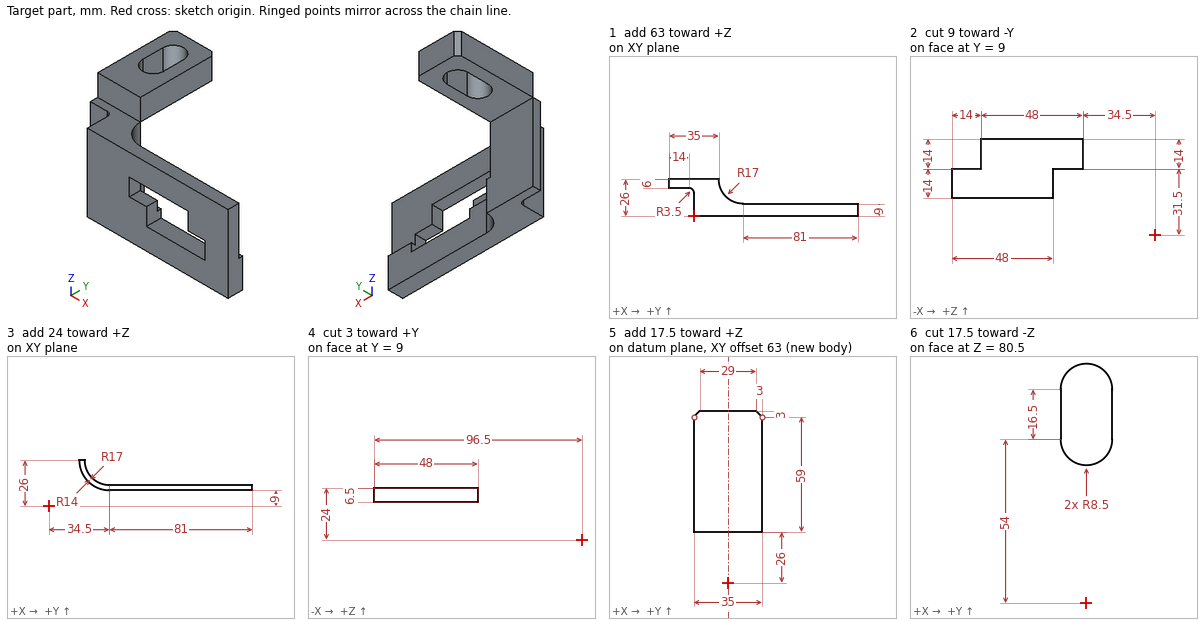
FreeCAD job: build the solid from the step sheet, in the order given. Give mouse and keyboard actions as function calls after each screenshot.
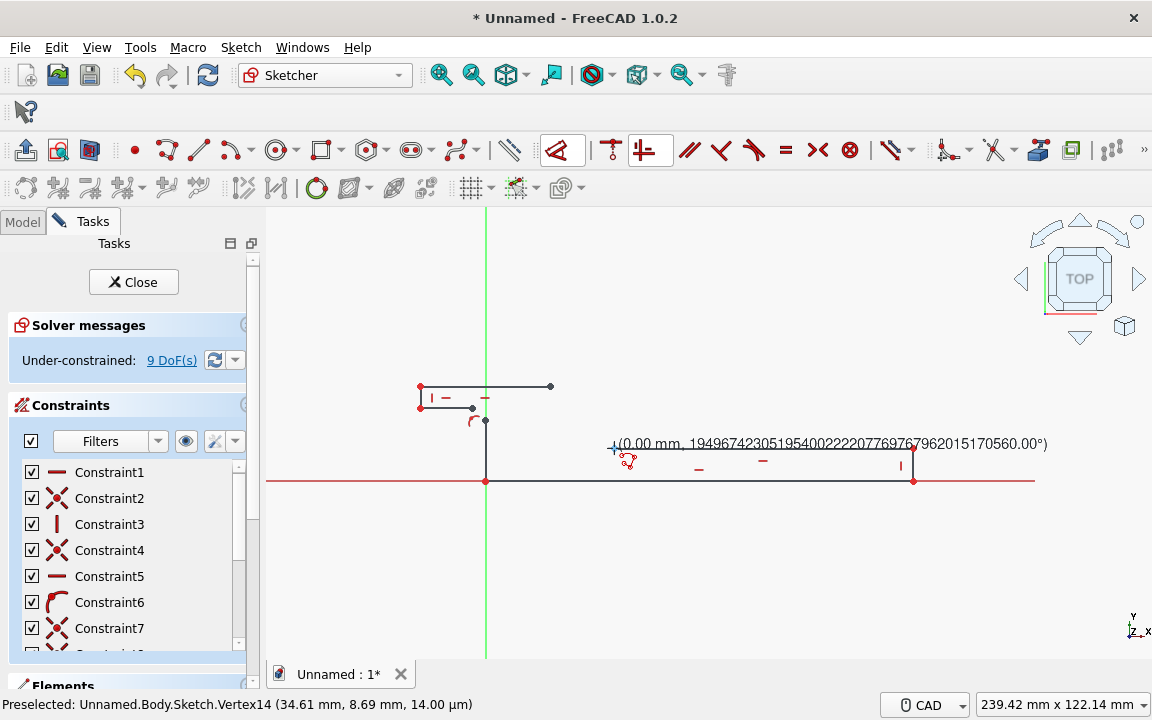
key(g)
key(3)
key(a)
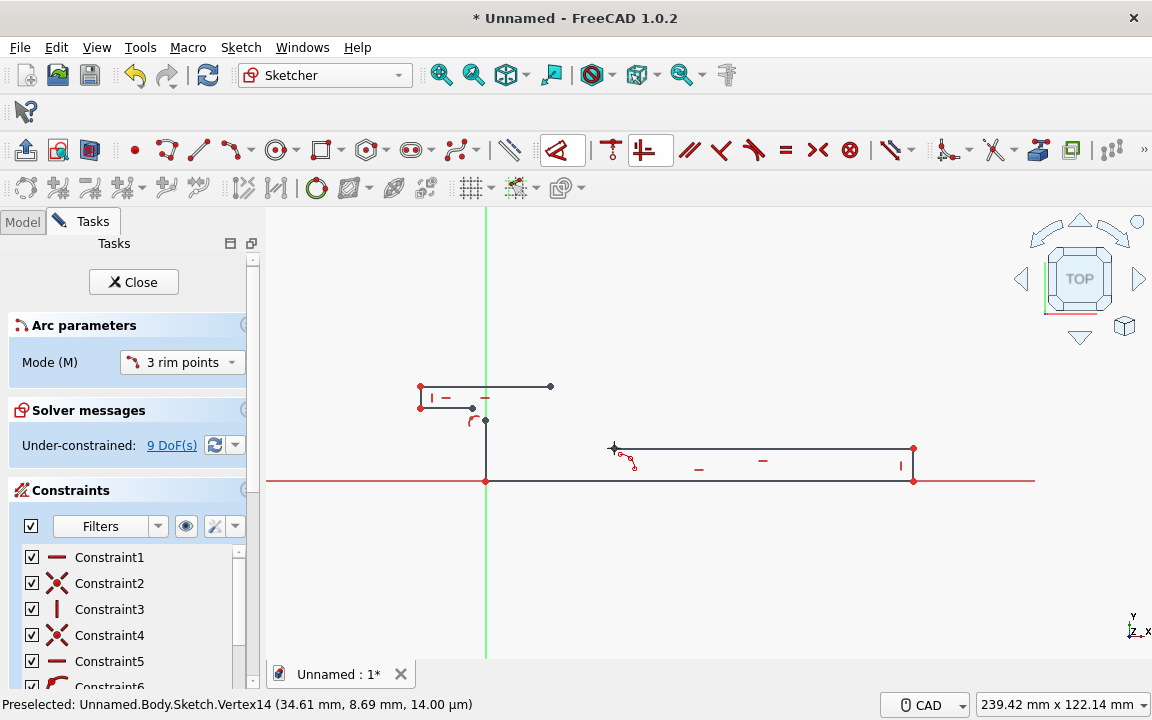
scroll(473, 407, up, 2)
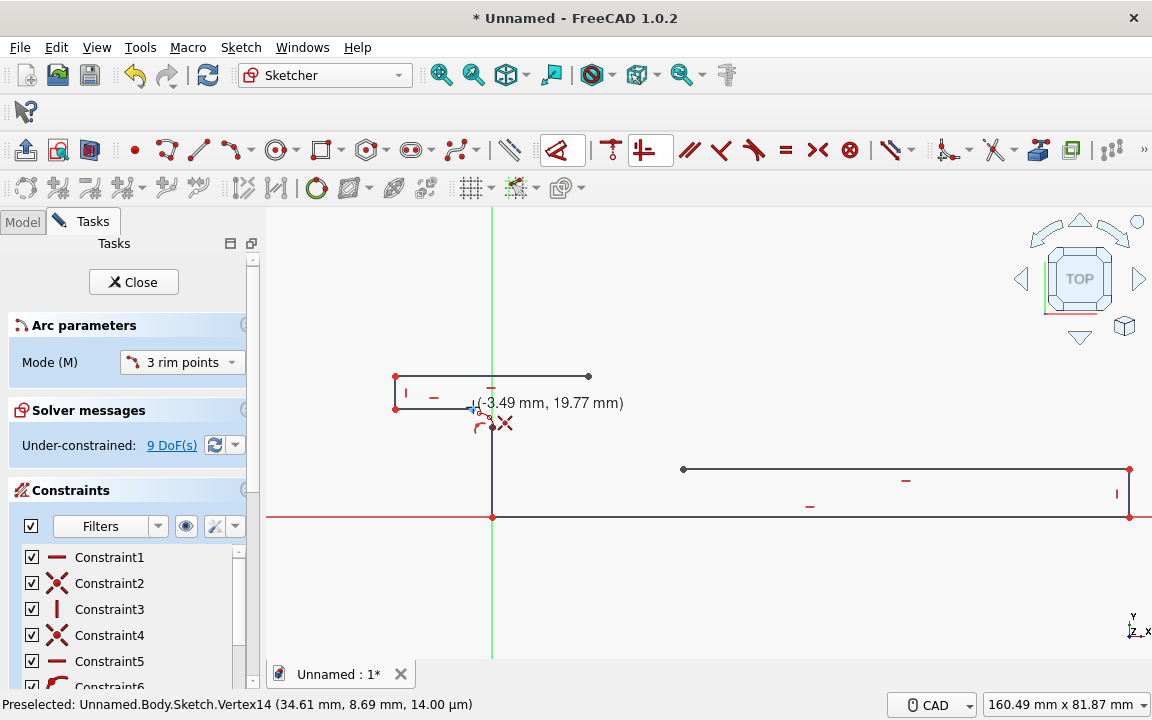
click(473, 409)
click(492, 428)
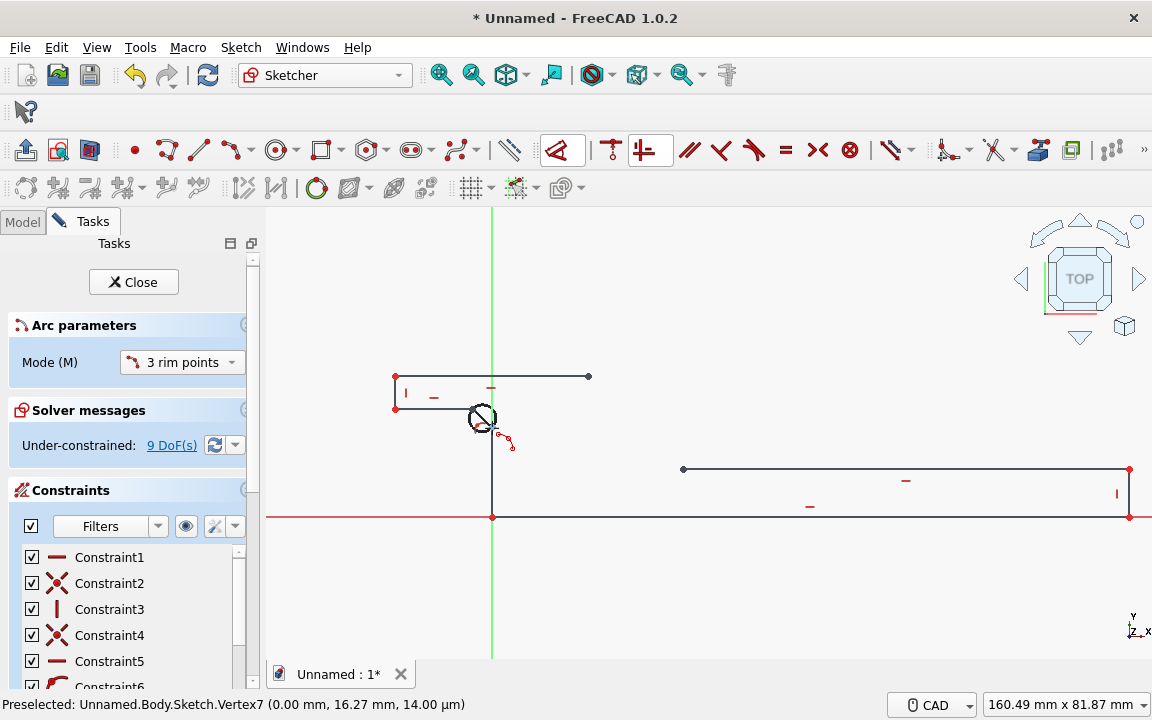
scroll(487, 413, up, 6)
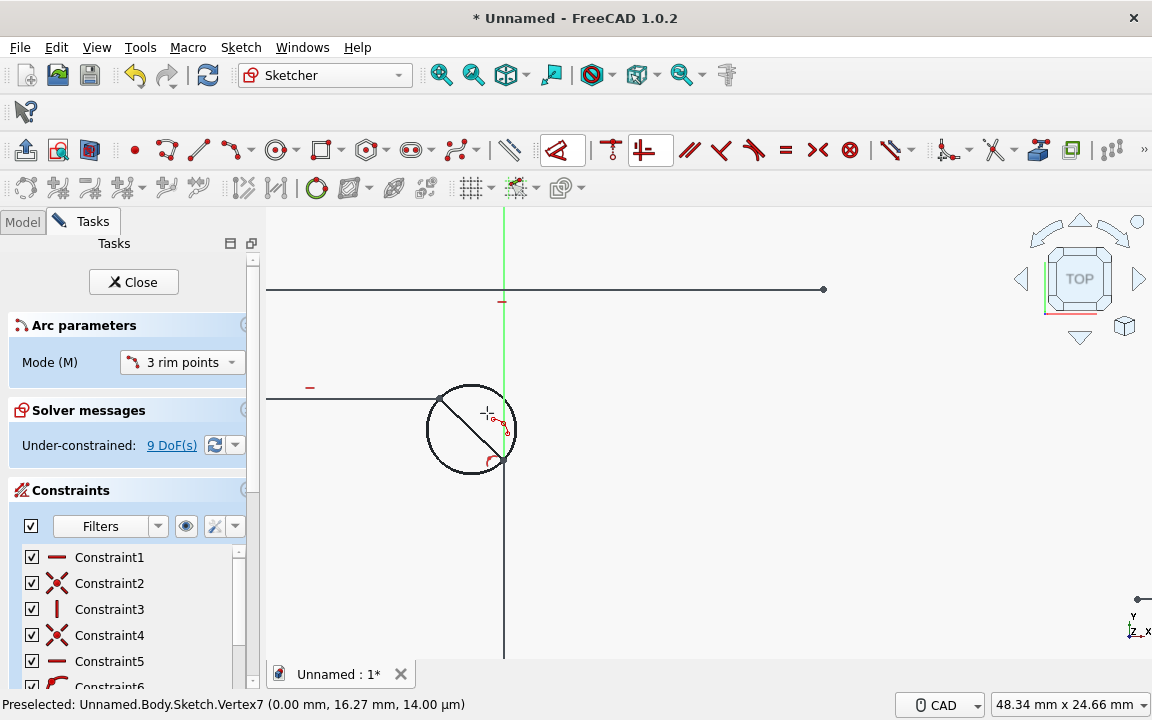
click(485, 411)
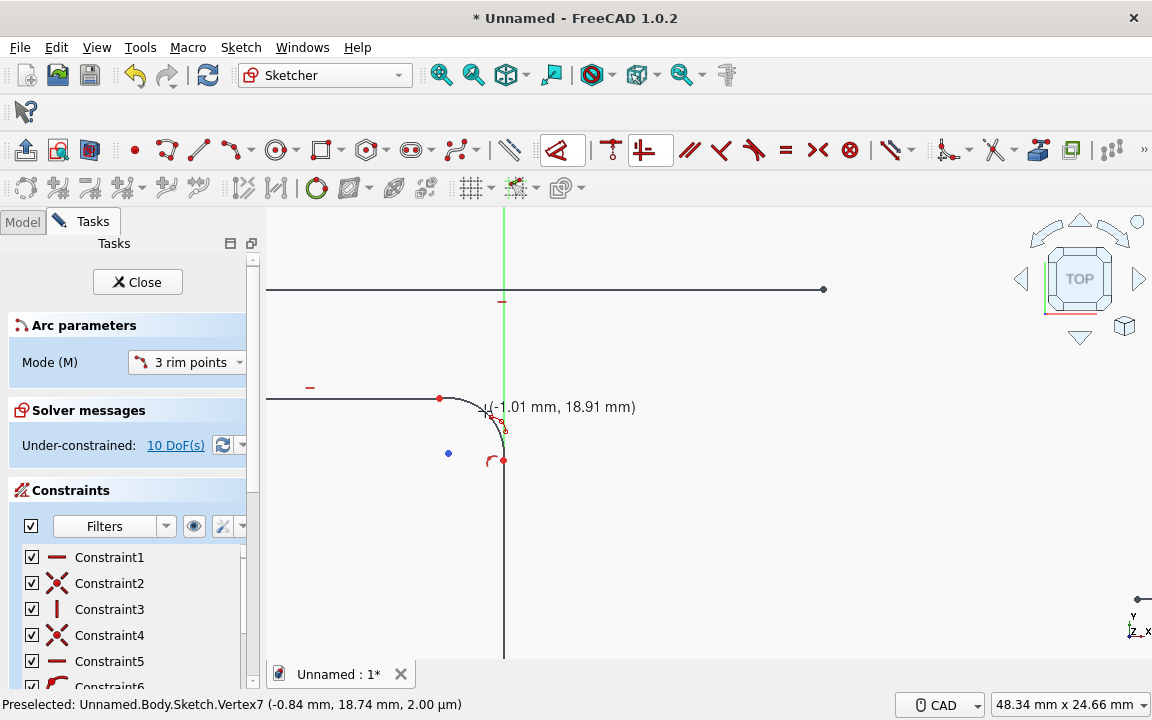
scroll(448, 411, down, 8)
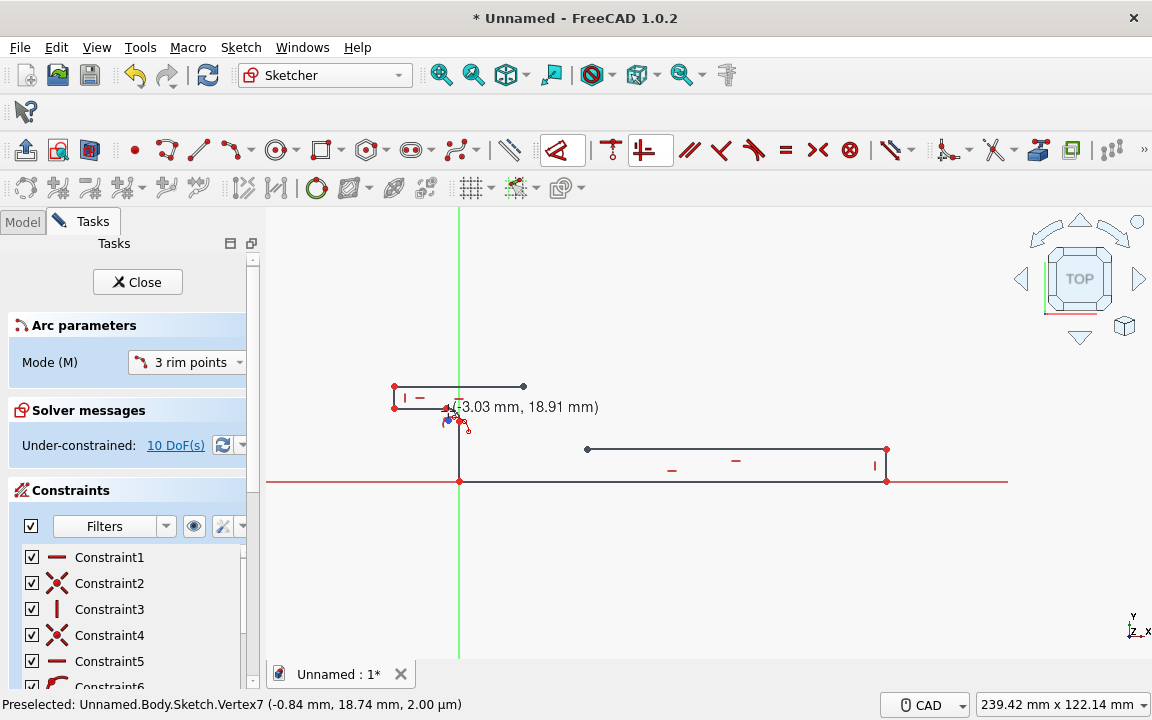
click(587, 449)
click(524, 387)
click(543, 430)
key(Escape)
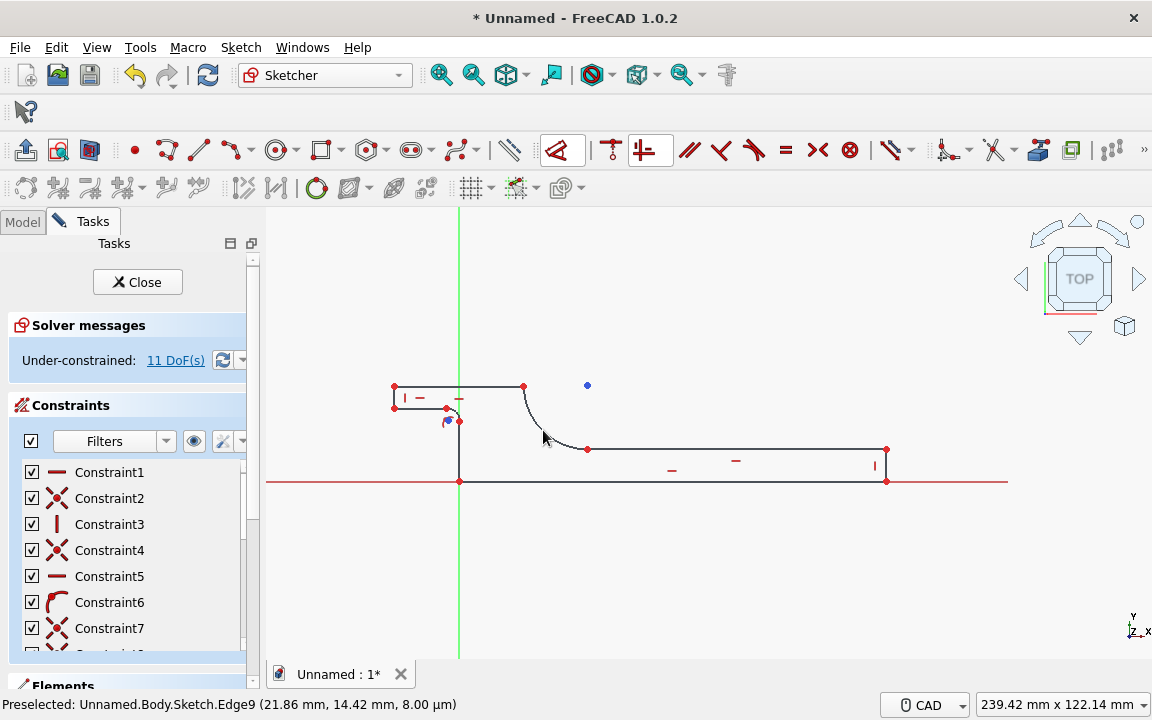
click(410, 409)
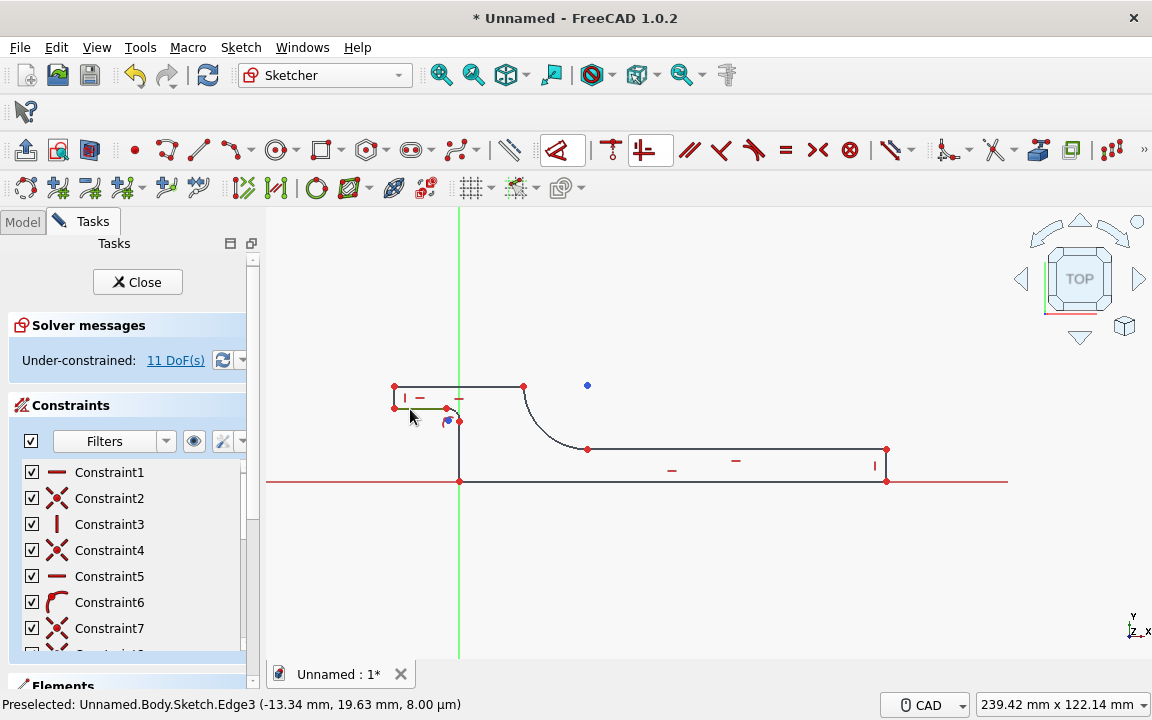
scroll(456, 412, up, 2)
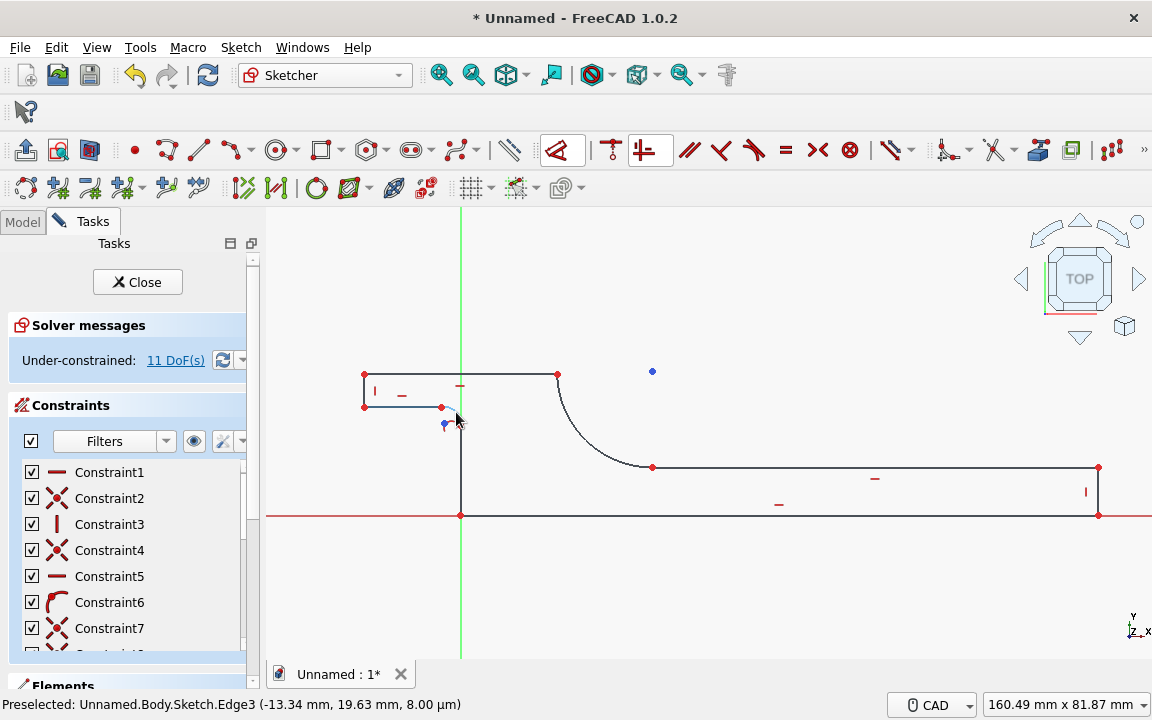
click(456, 412)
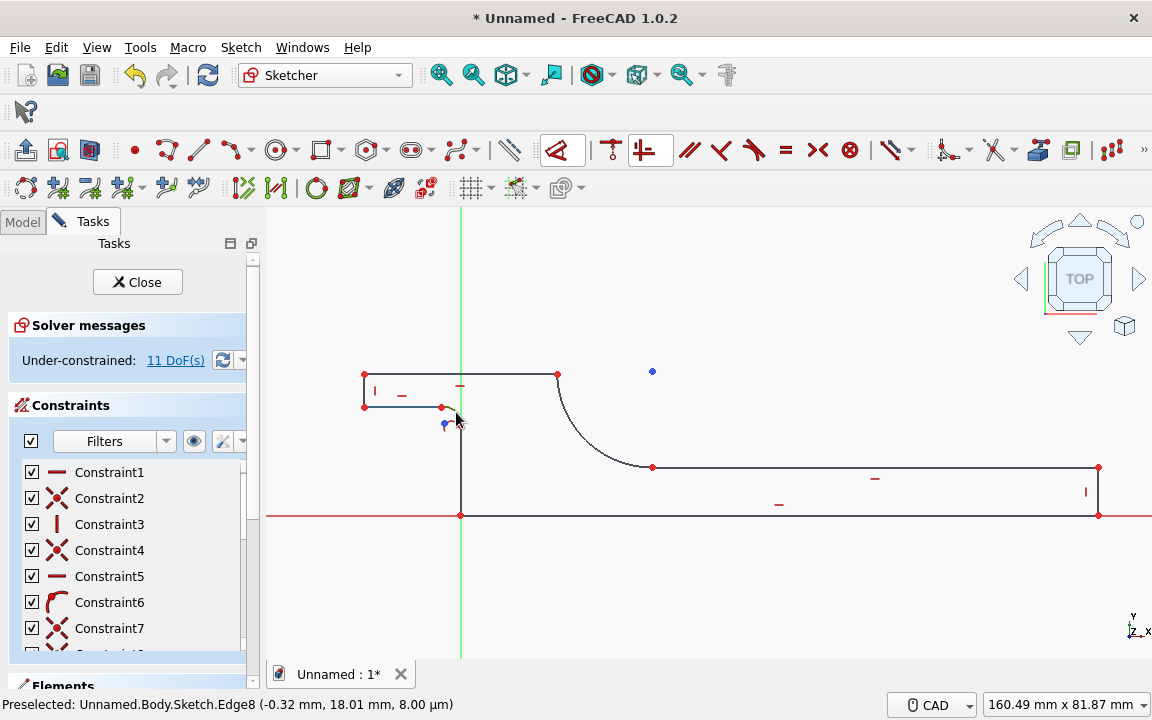
click(754, 150)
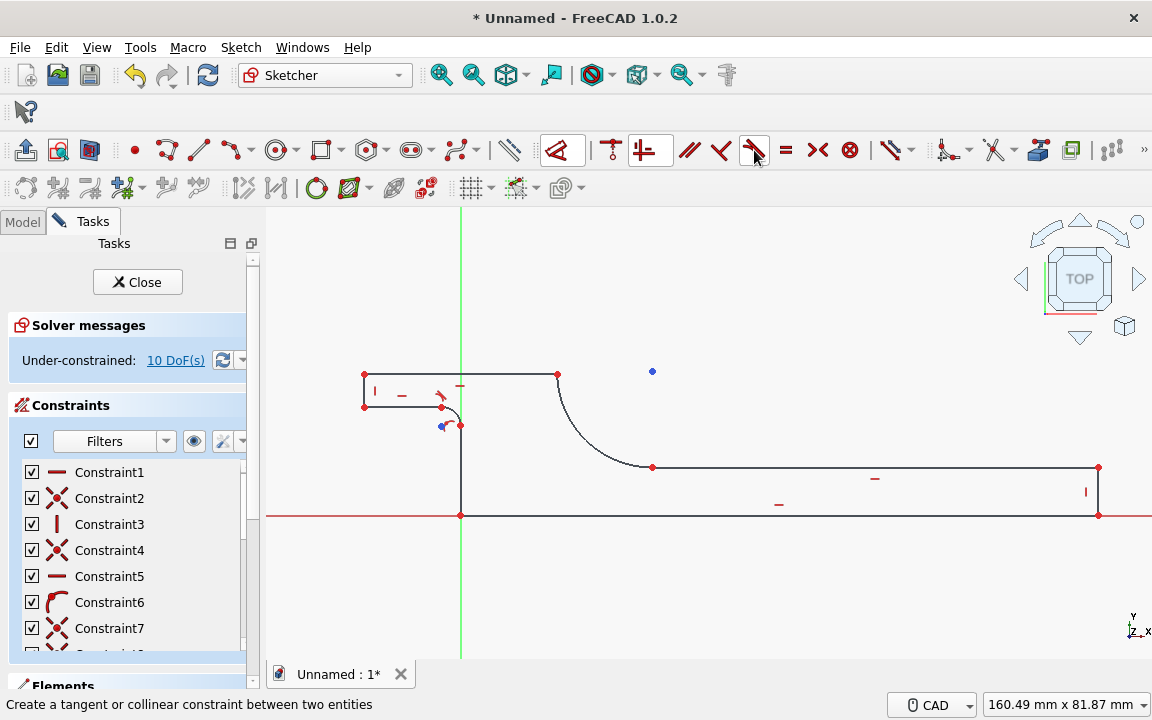
click(461, 453)